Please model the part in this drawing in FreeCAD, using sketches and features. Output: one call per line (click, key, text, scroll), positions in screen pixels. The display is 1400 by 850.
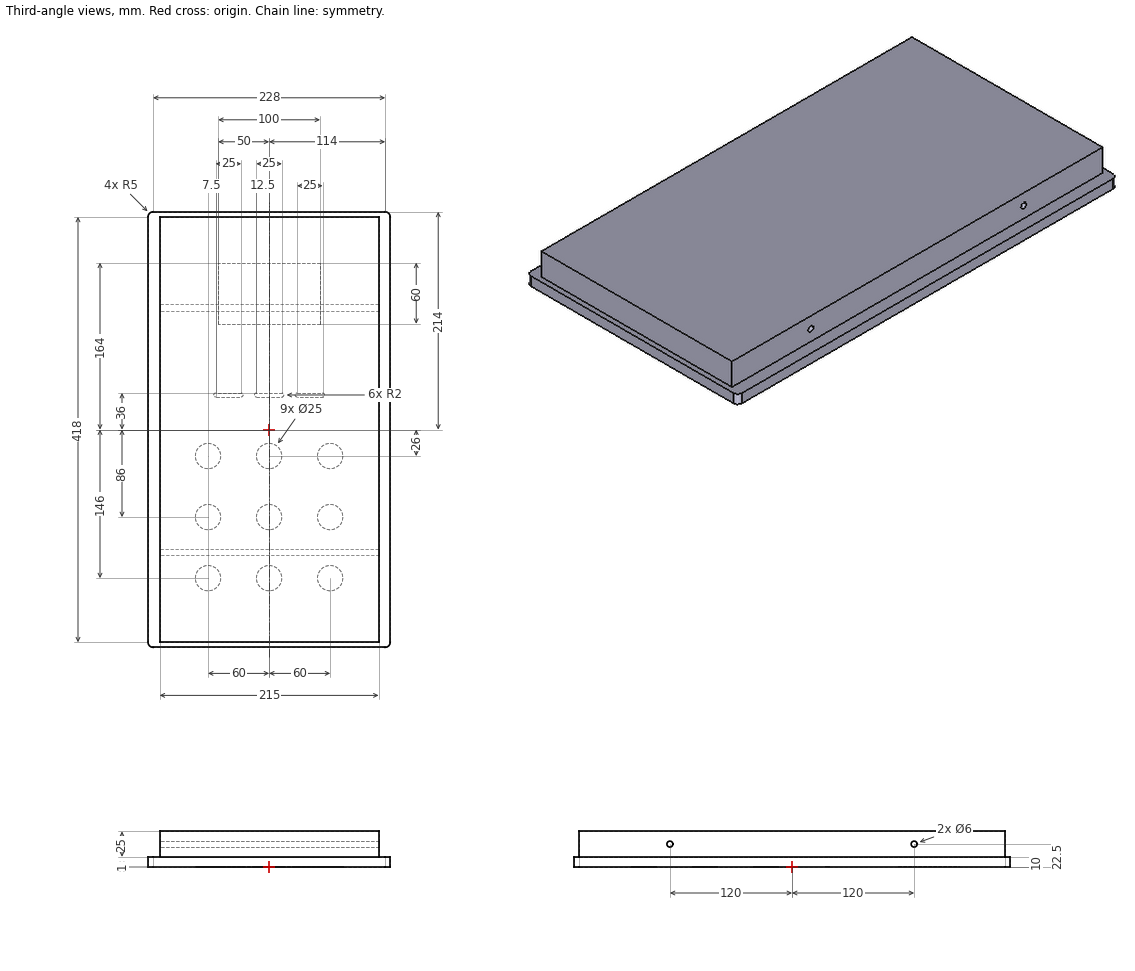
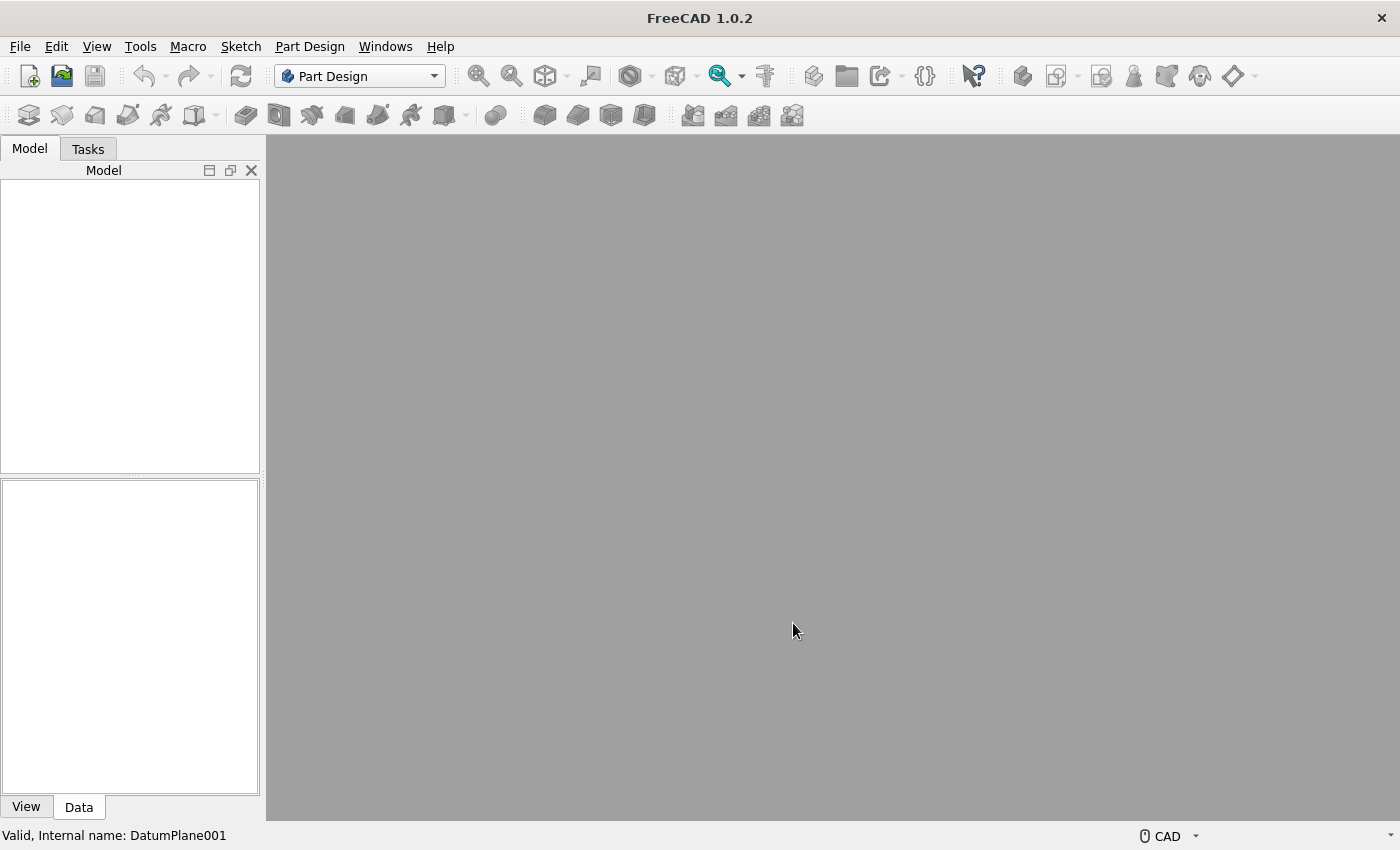
key(ctrl+n)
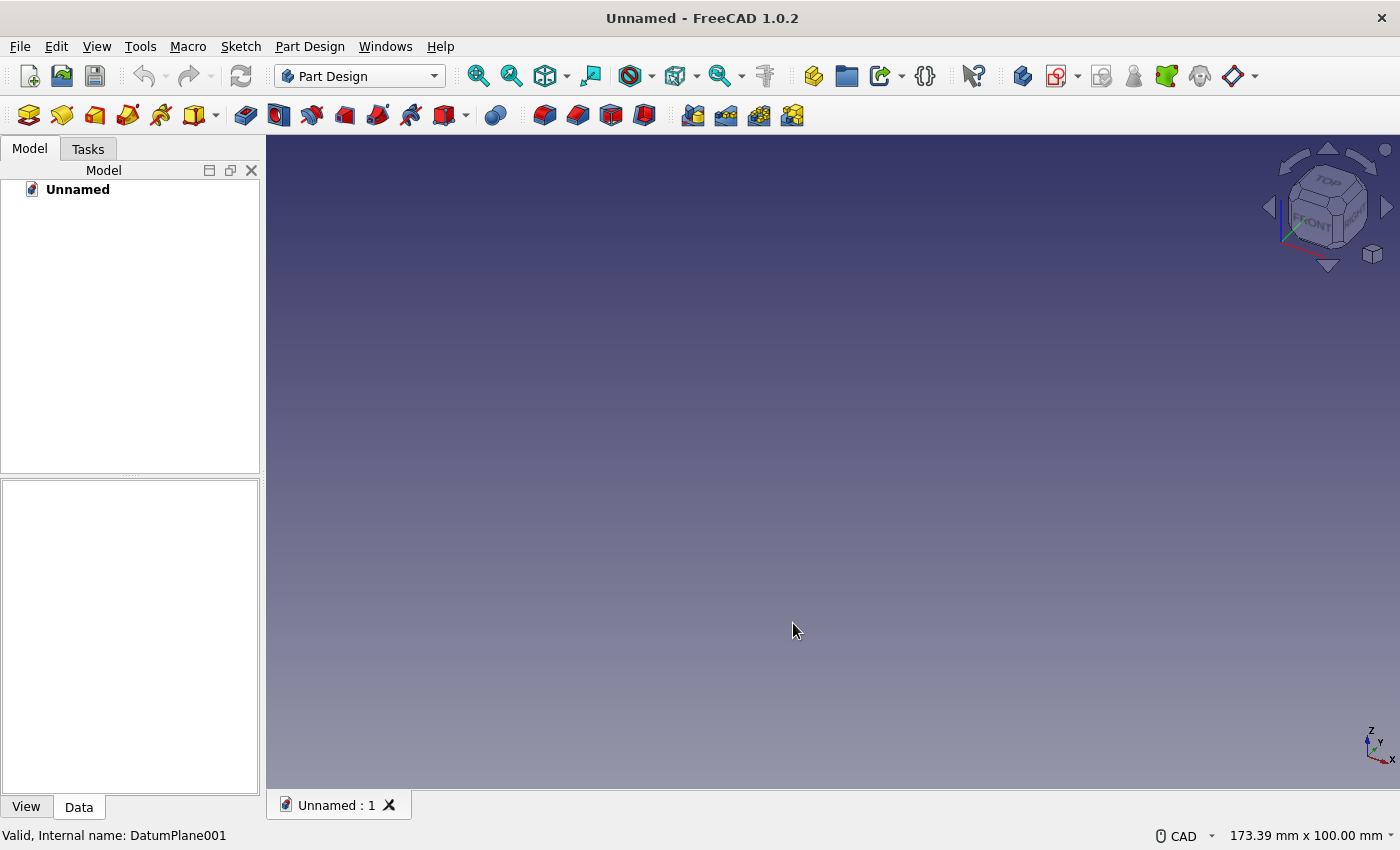
click(1056, 76)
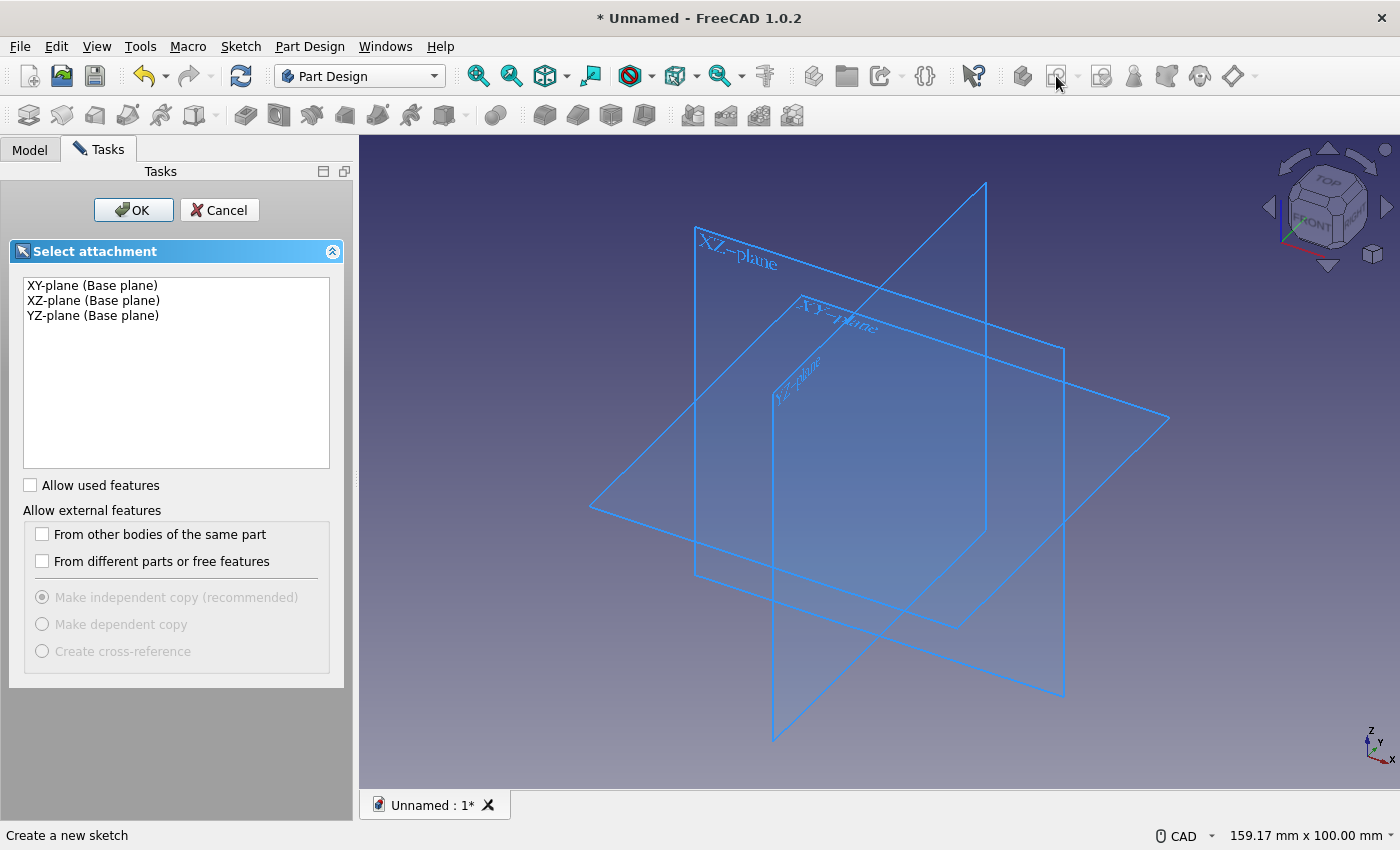
click(84, 286)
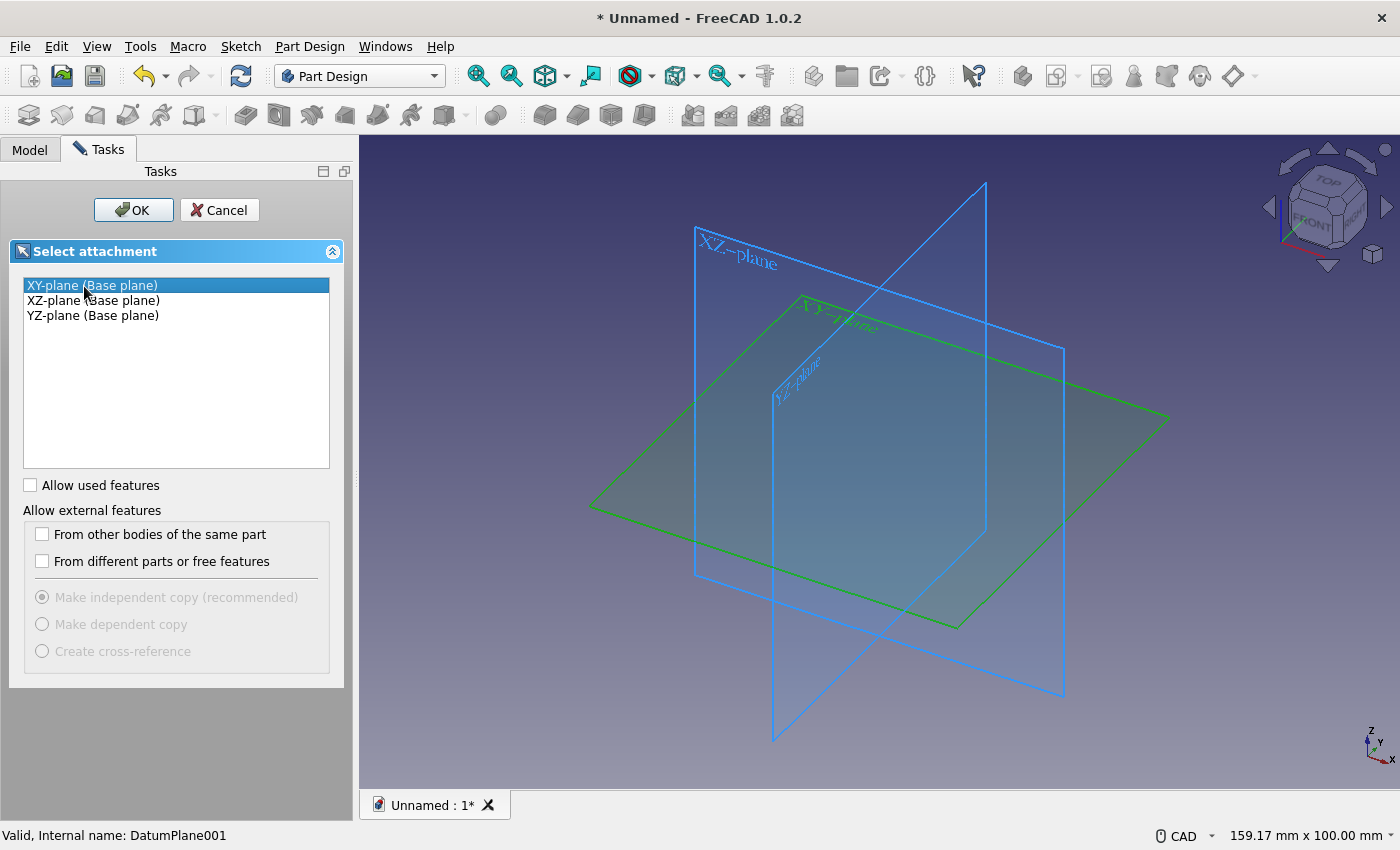
click(134, 210)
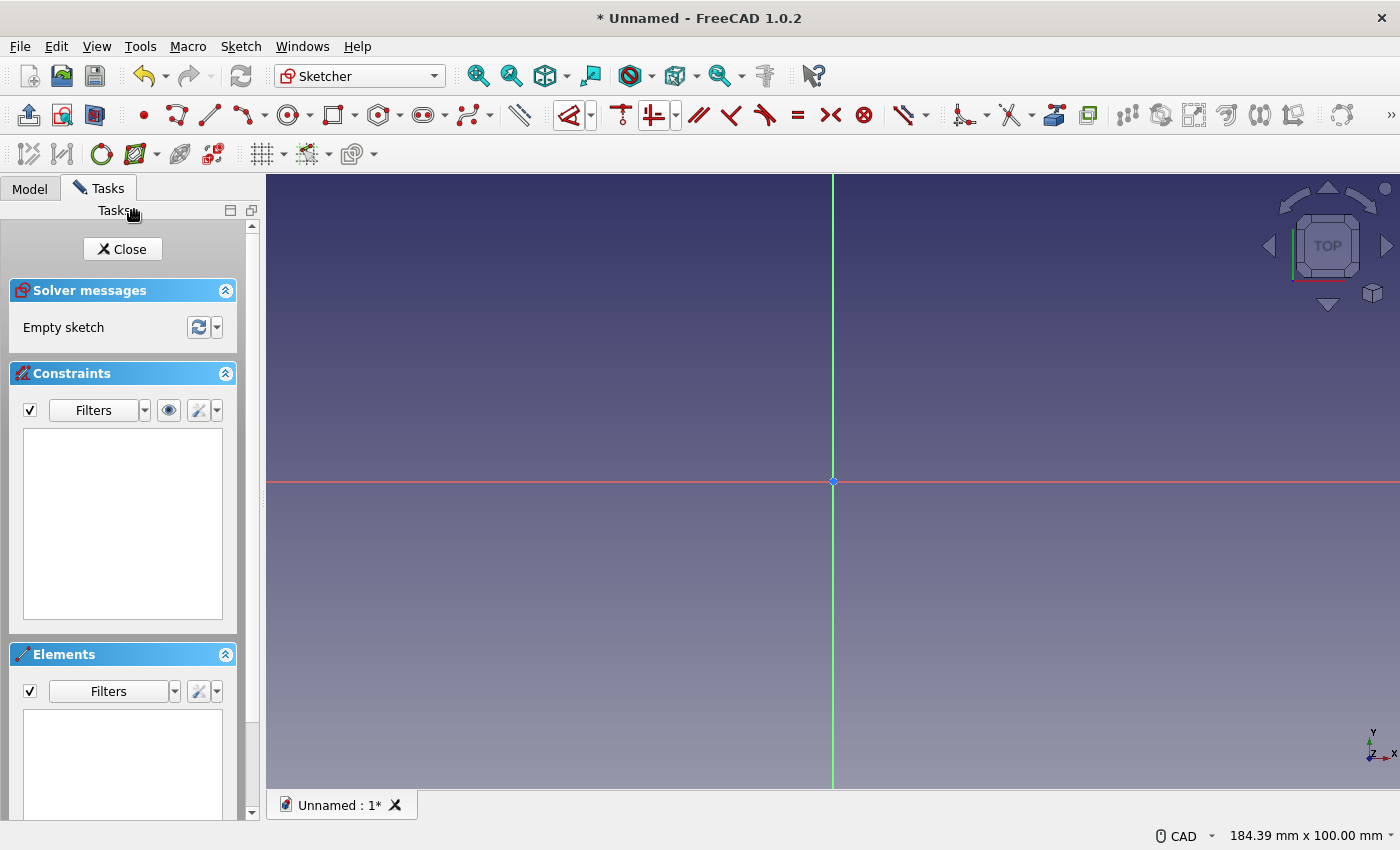
scroll(751, 482, down, 9)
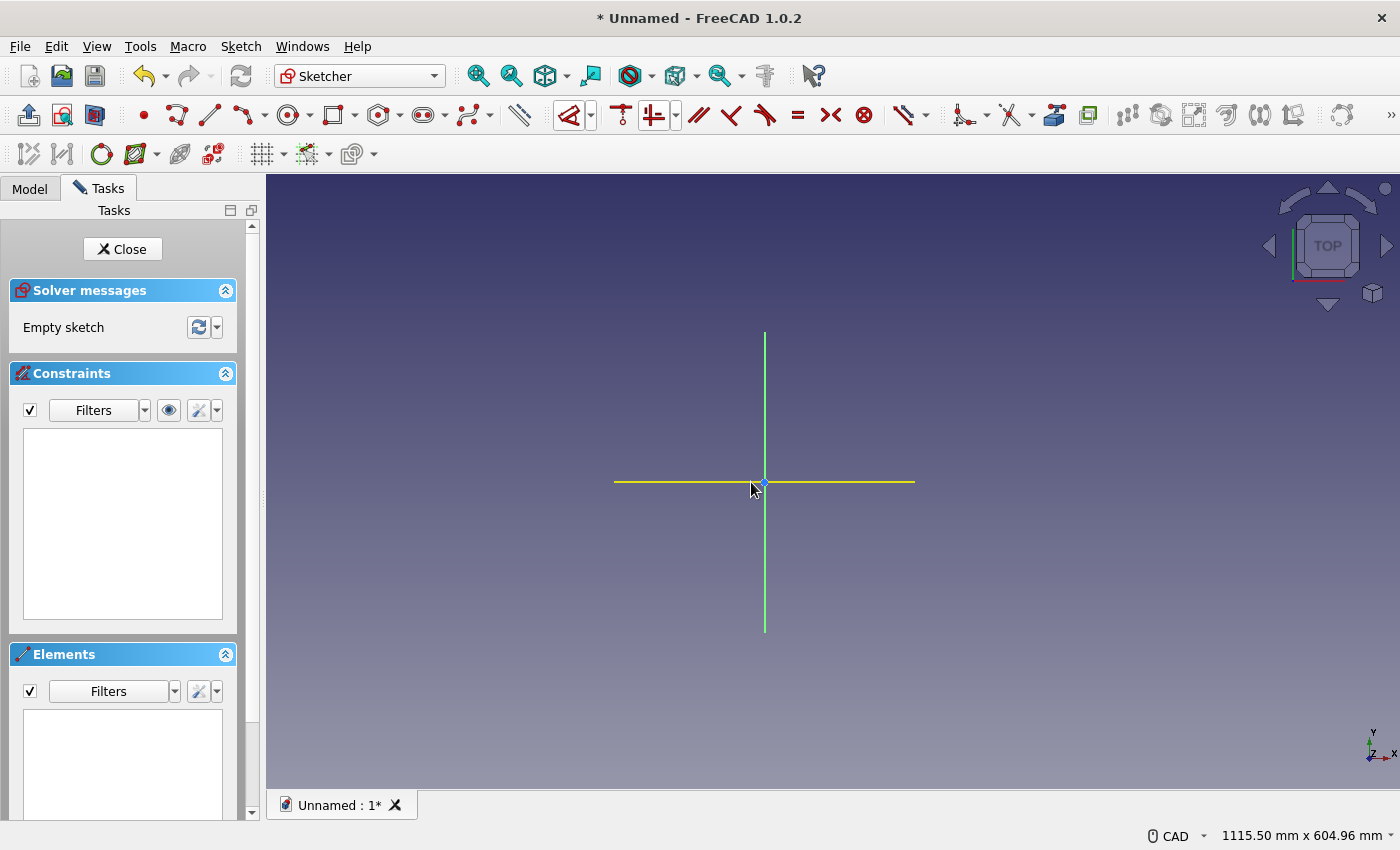
click(210, 116)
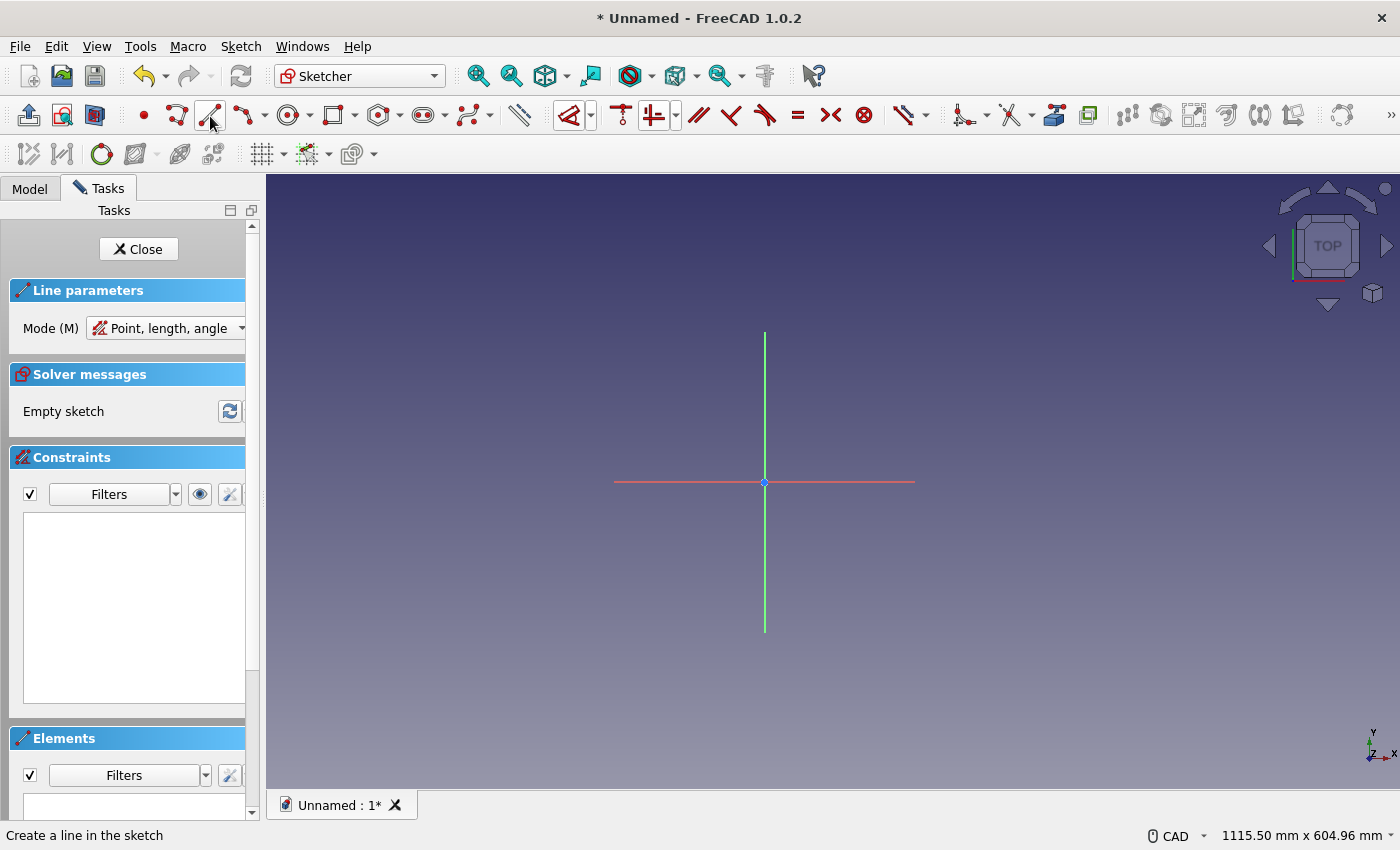
click(881, 265)
click(649, 265)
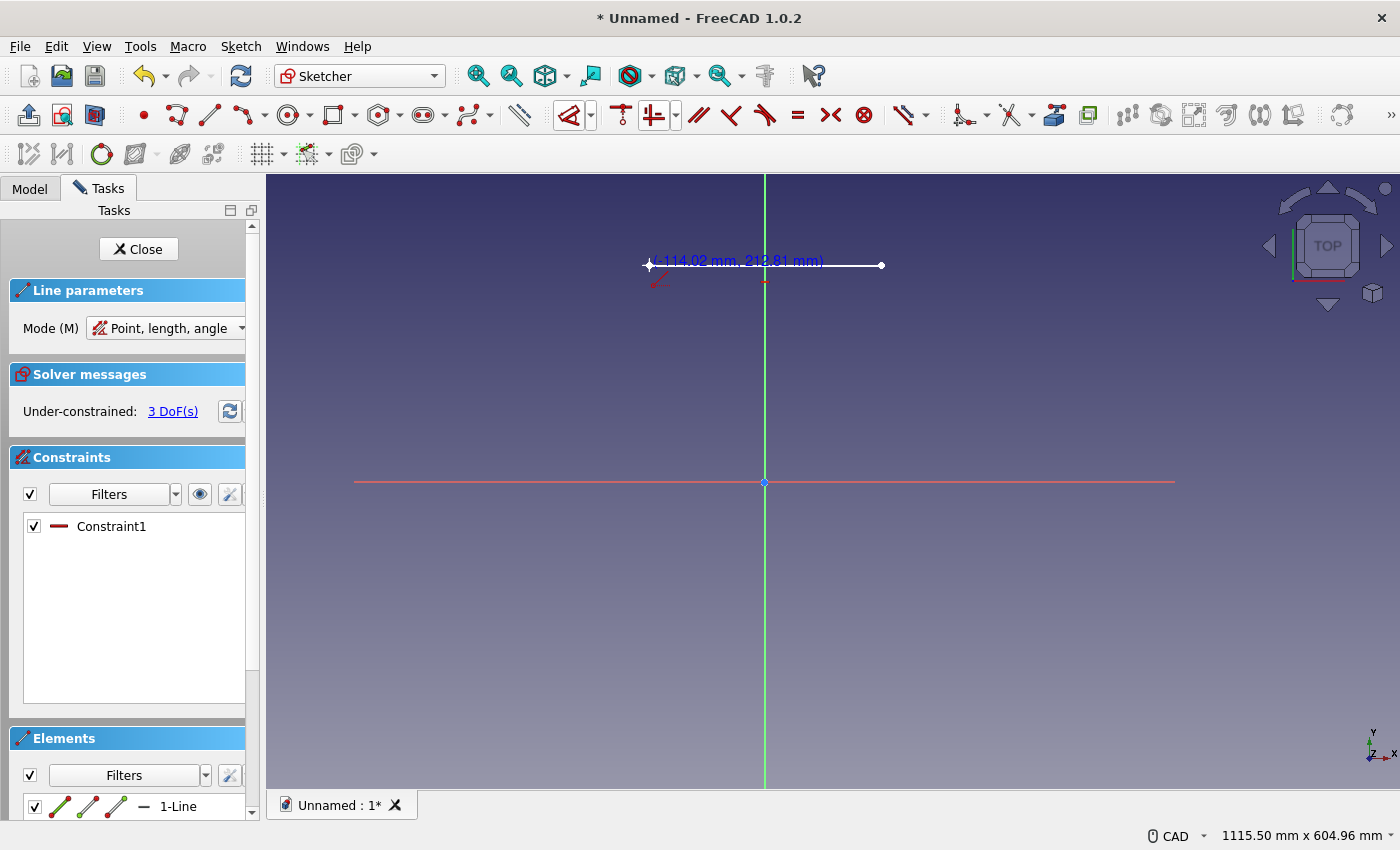
scroll(644, 270, up, 4)